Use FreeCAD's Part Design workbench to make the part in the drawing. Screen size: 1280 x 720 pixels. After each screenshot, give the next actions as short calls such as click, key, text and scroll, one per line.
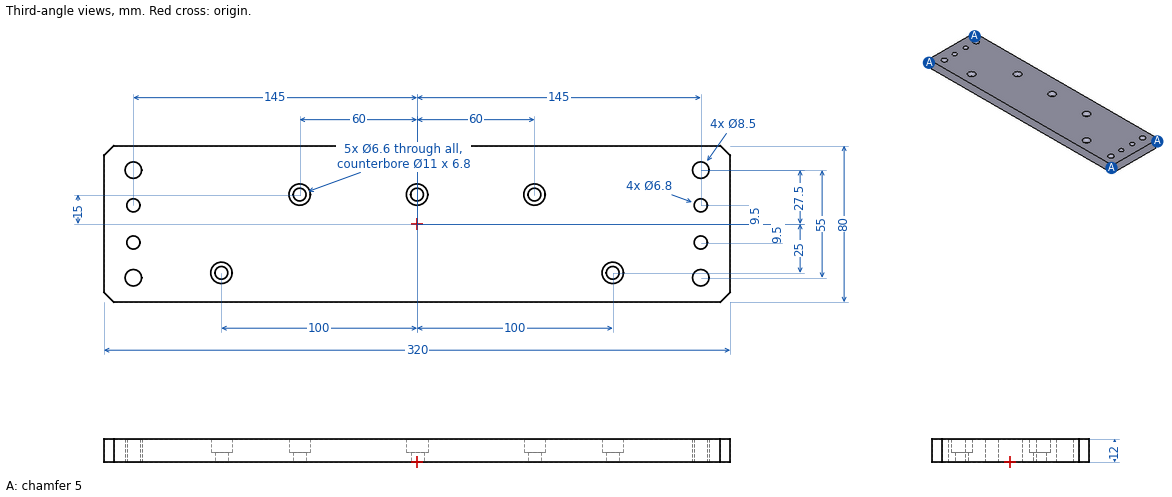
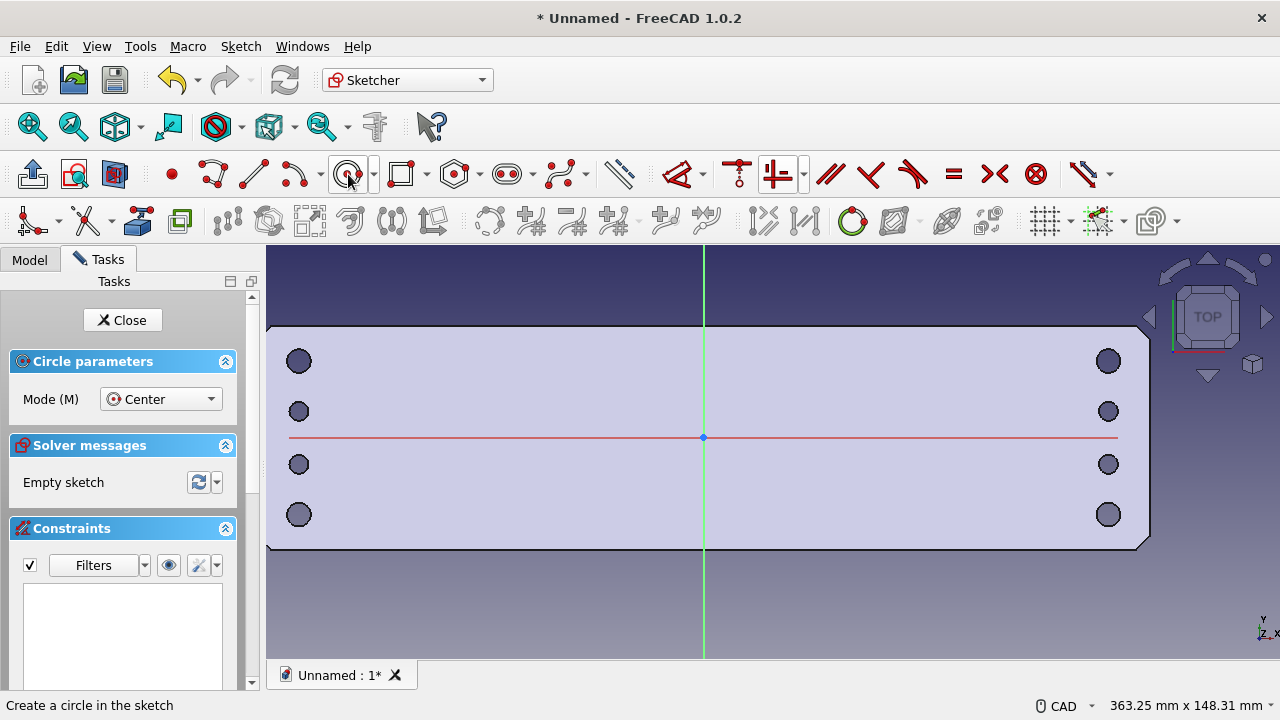
scroll(536, 396, up, 5)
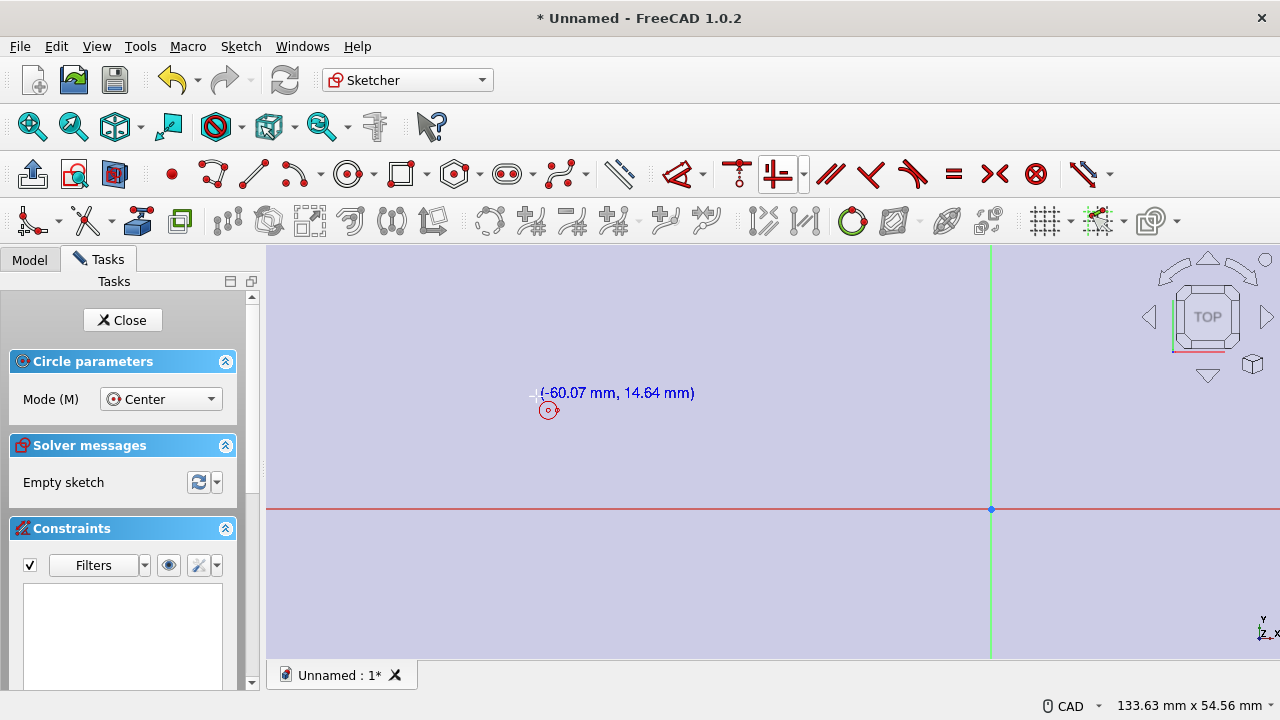
click(536, 395)
click(554, 378)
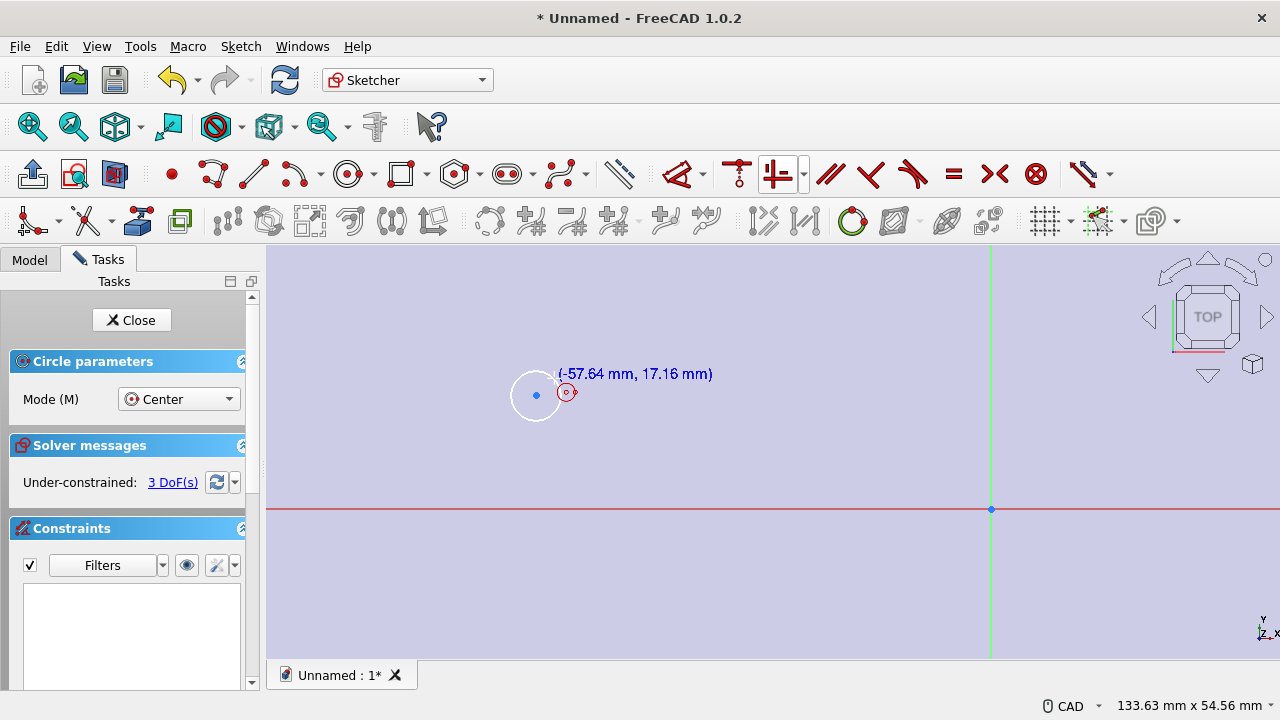
click(991, 395)
click(1009, 378)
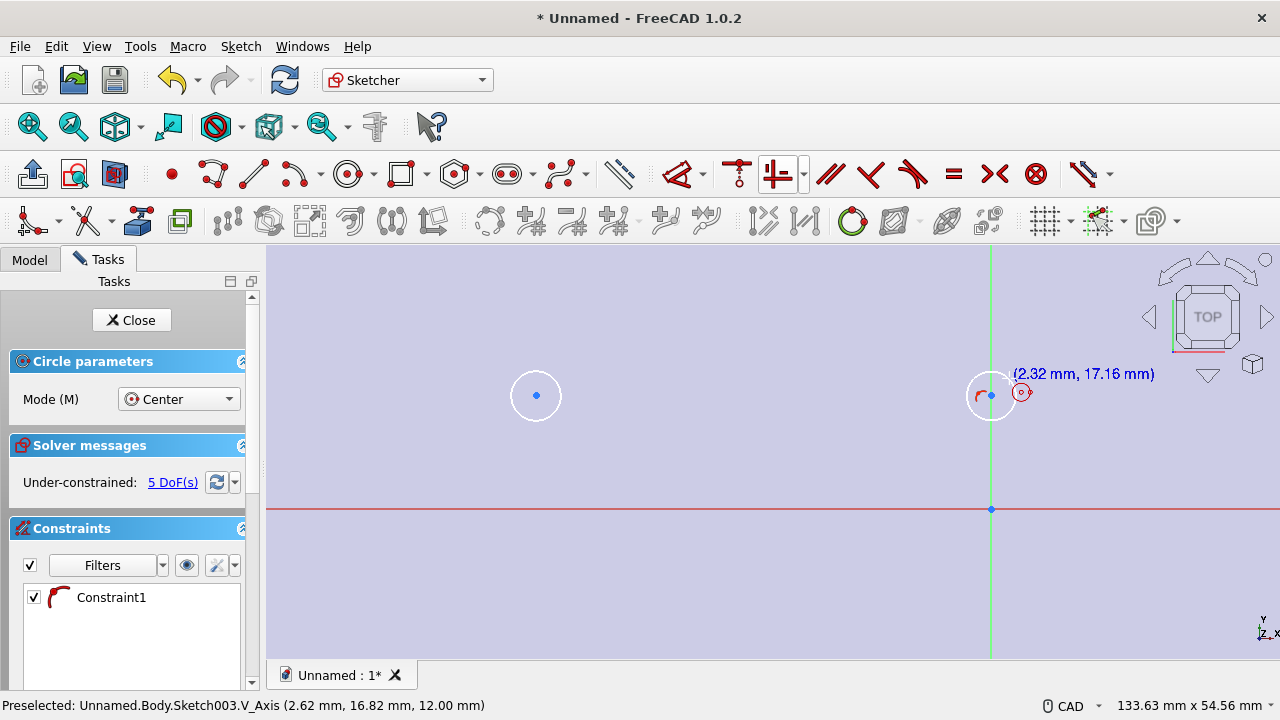
scroll(538, 397, down, 5)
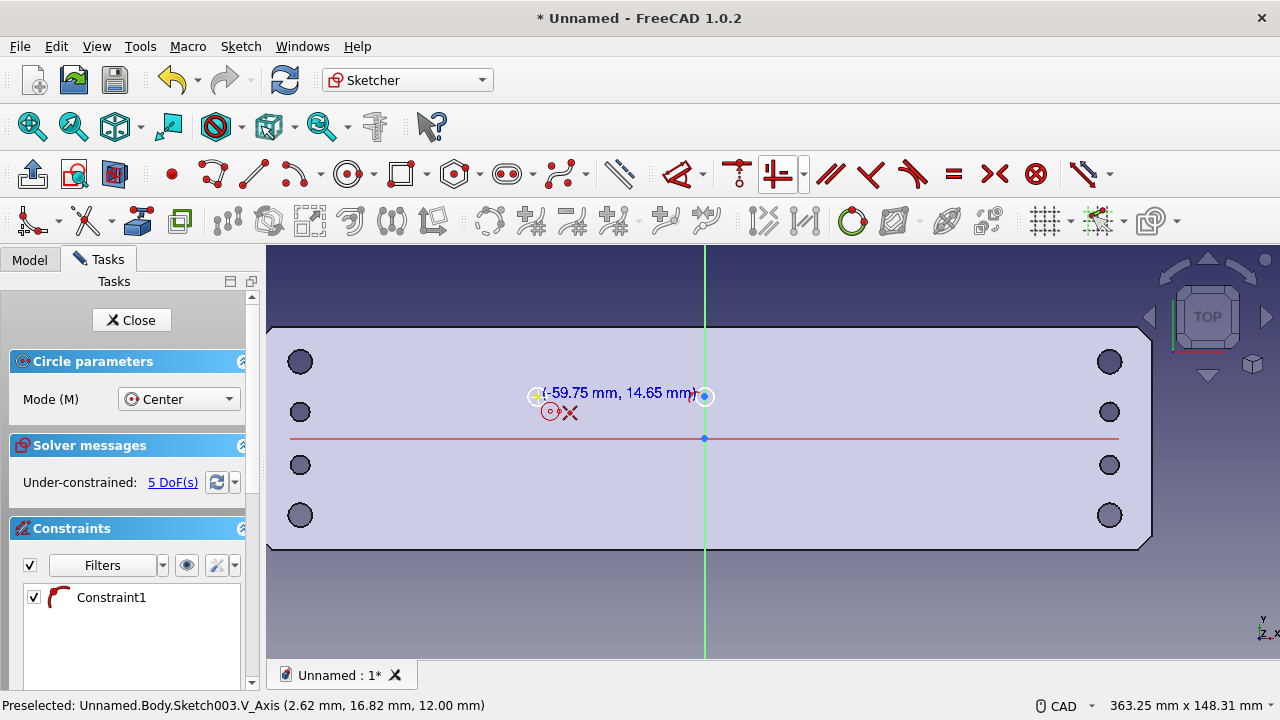
scroll(872, 397, up, 5)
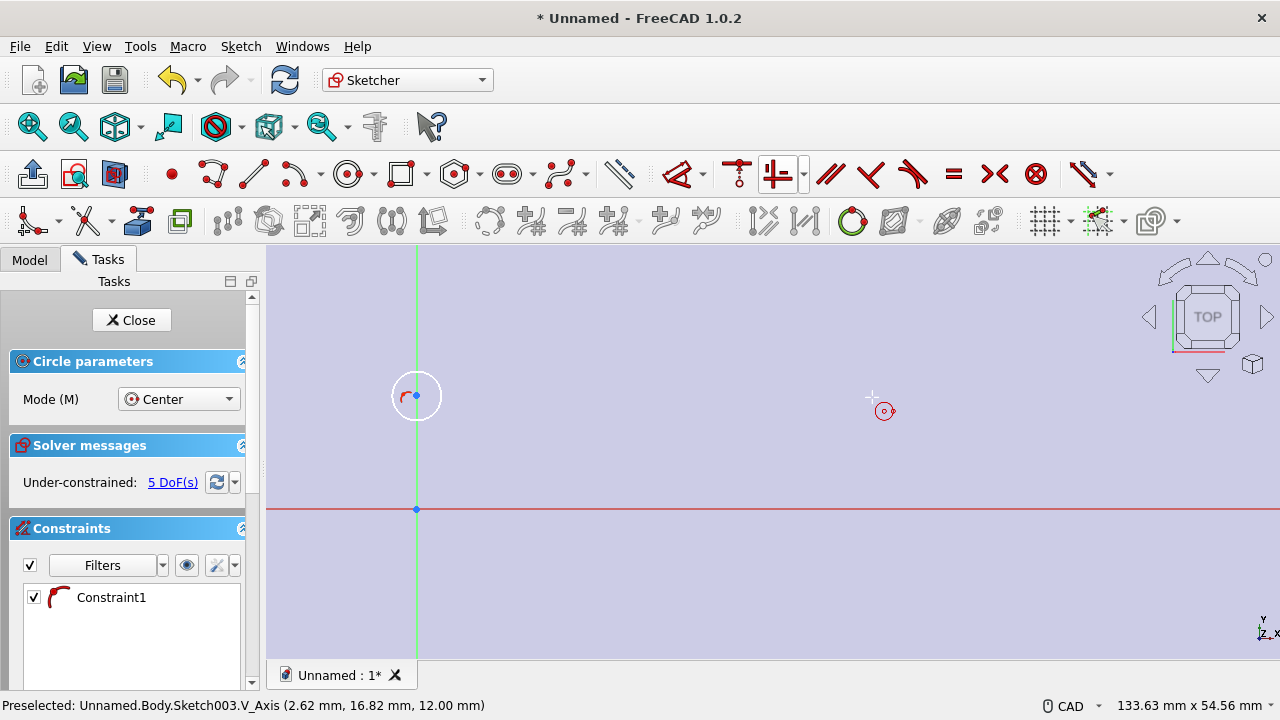
click(872, 395)
click(890, 378)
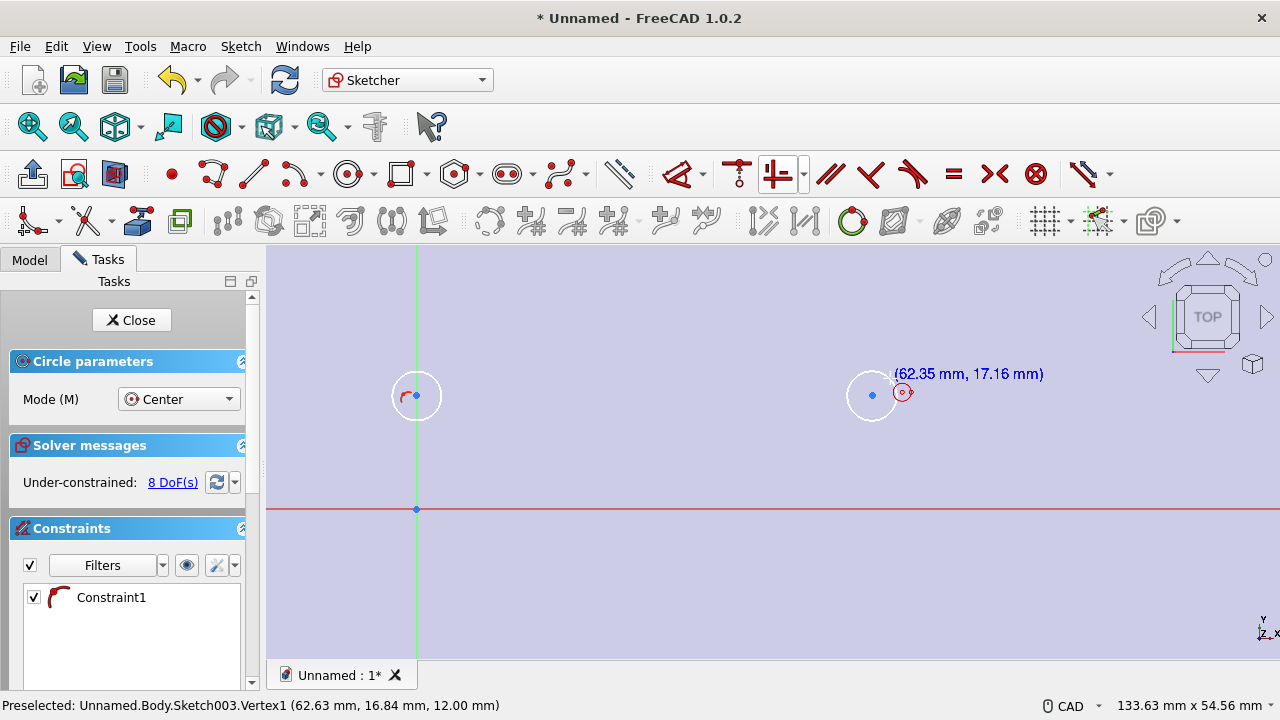
scroll(872, 397, down, 5)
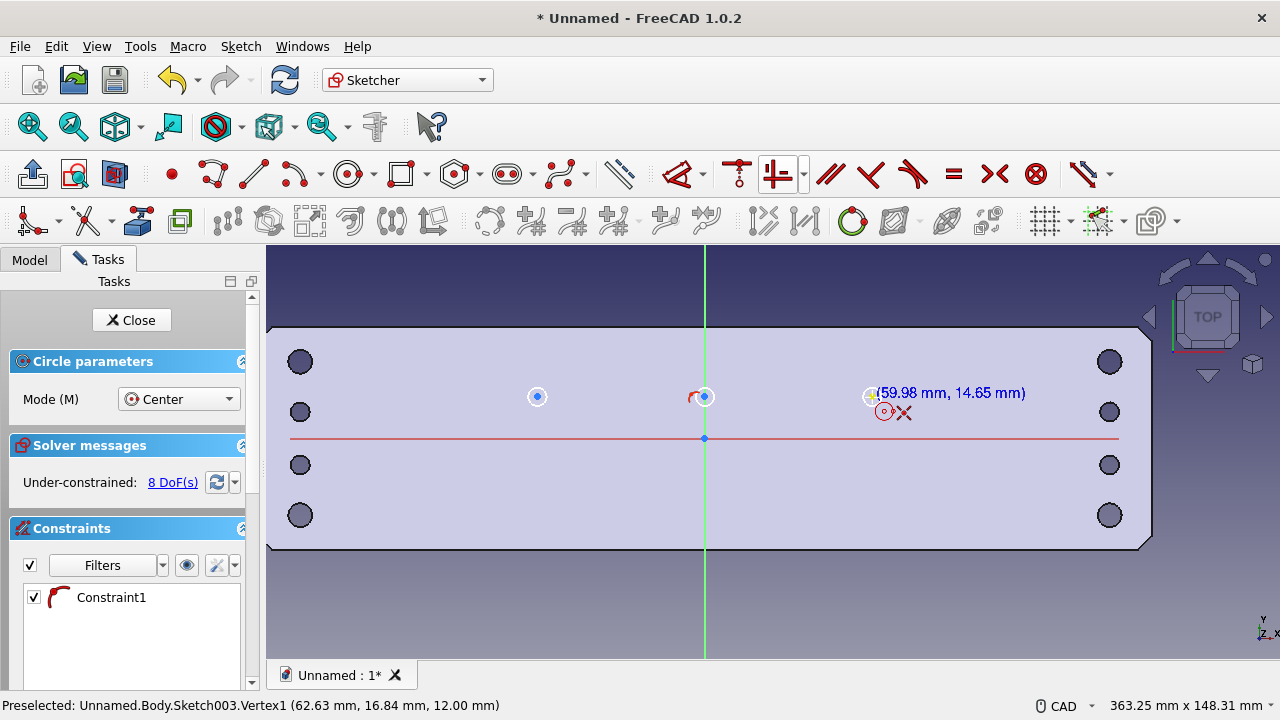
scroll(984, 508, up, 5)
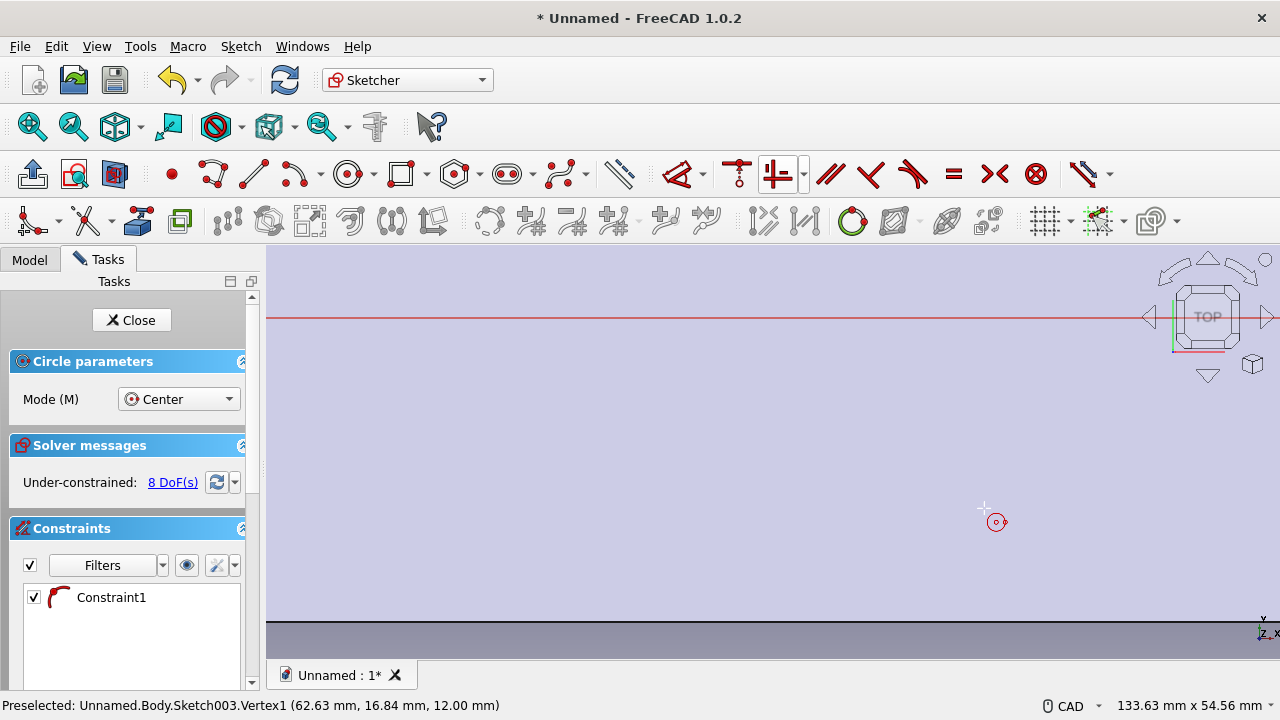
click(983, 508)
click(1001, 490)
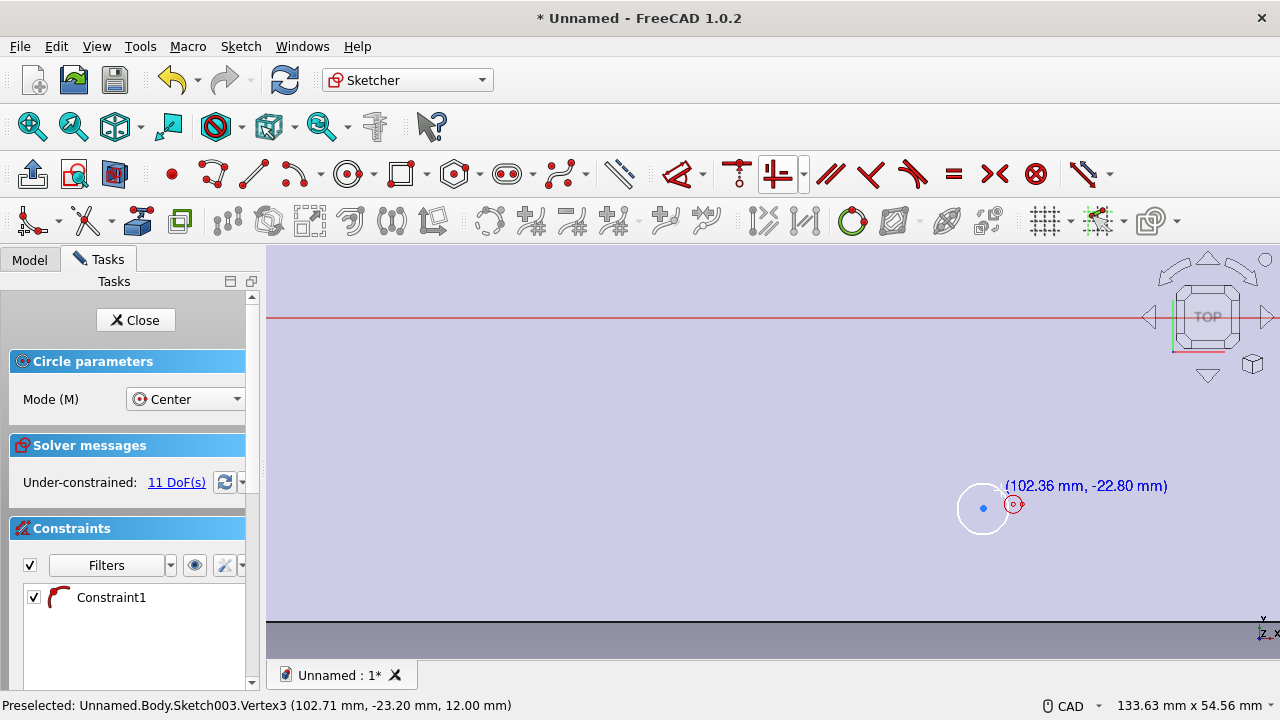
scroll(984, 508, down, 5)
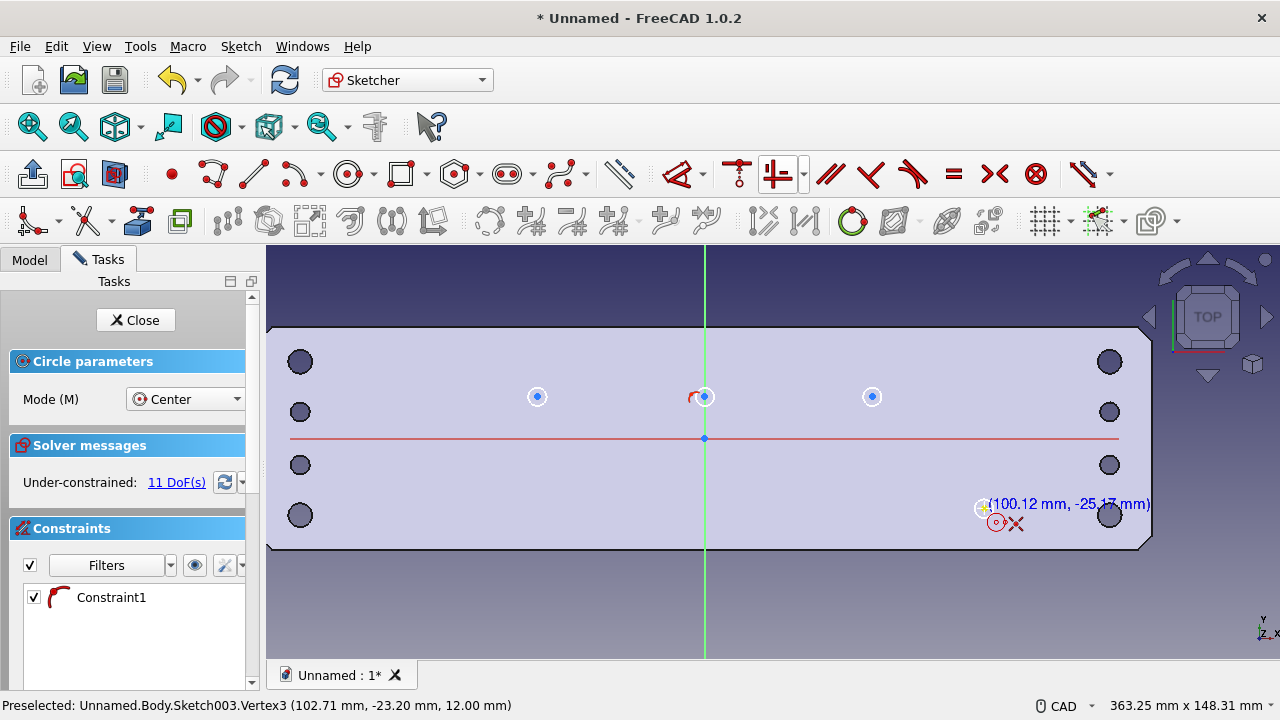
scroll(426, 508, up, 5)